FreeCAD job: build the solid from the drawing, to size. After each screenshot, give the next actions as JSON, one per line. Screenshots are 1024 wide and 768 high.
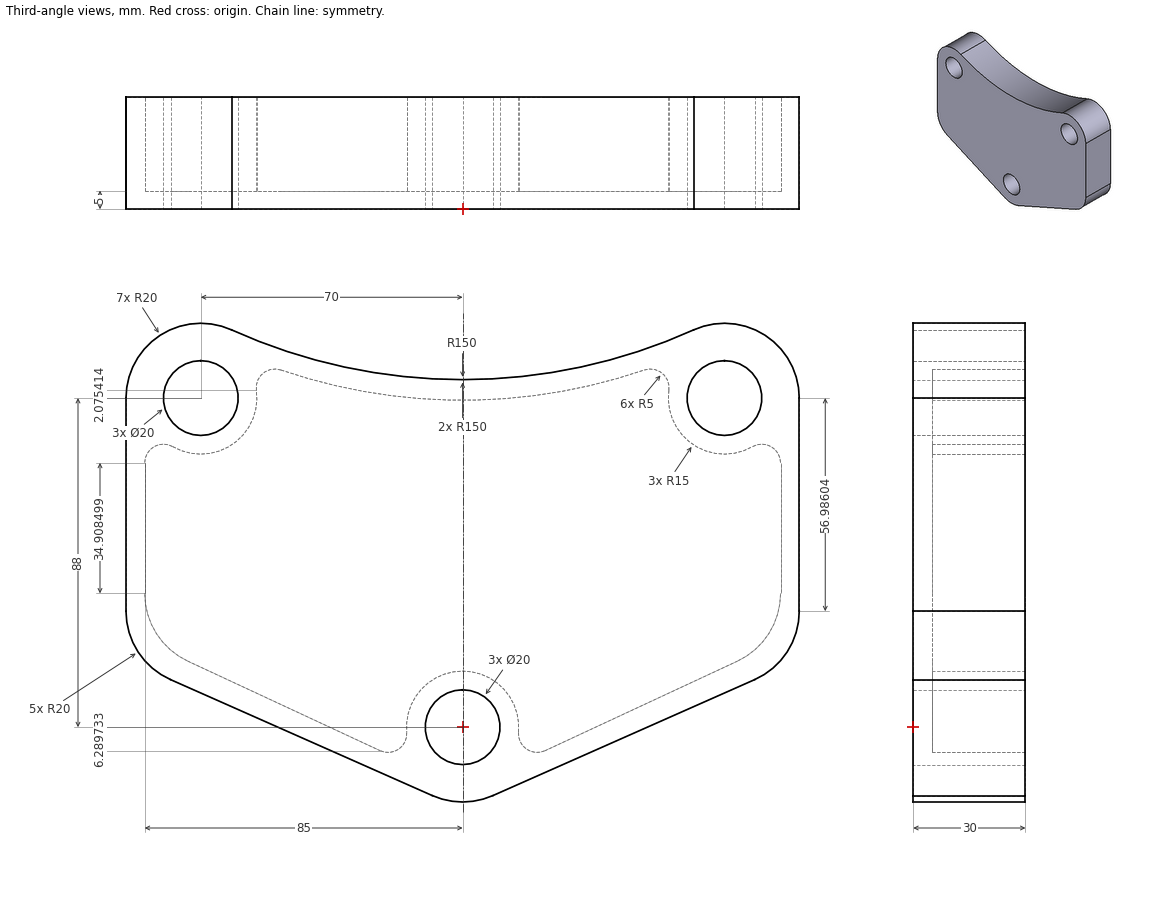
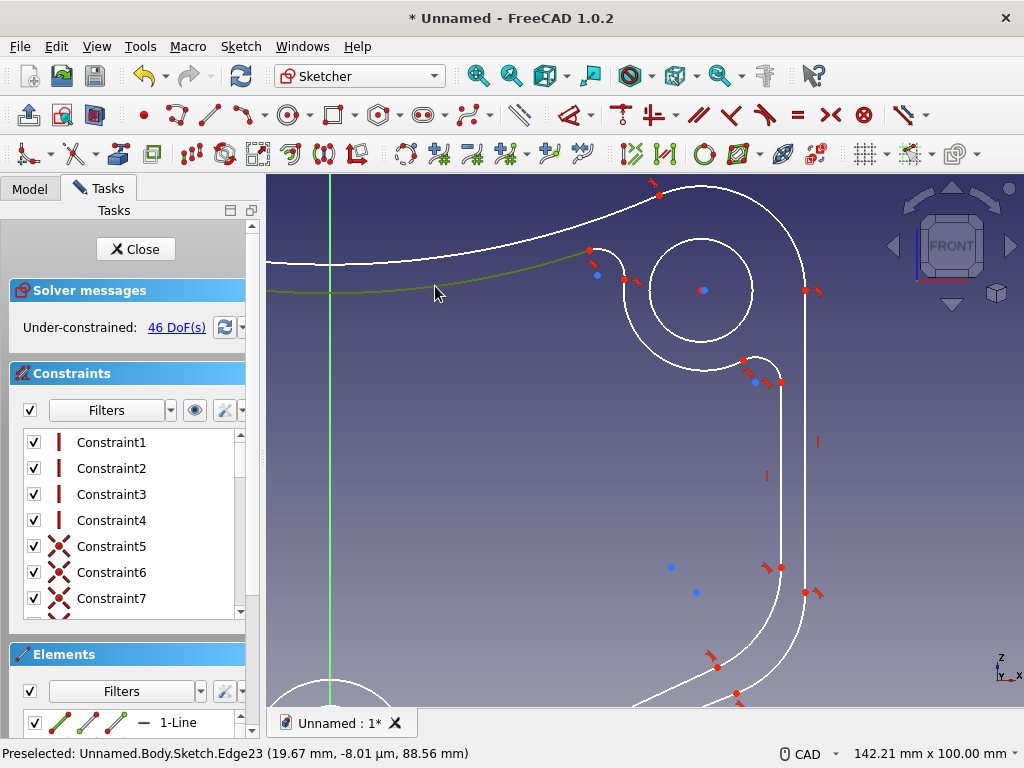
{"action": "scroll", "coordinate": [777, 369], "scroll_direction": "down", "scroll_amount": 4}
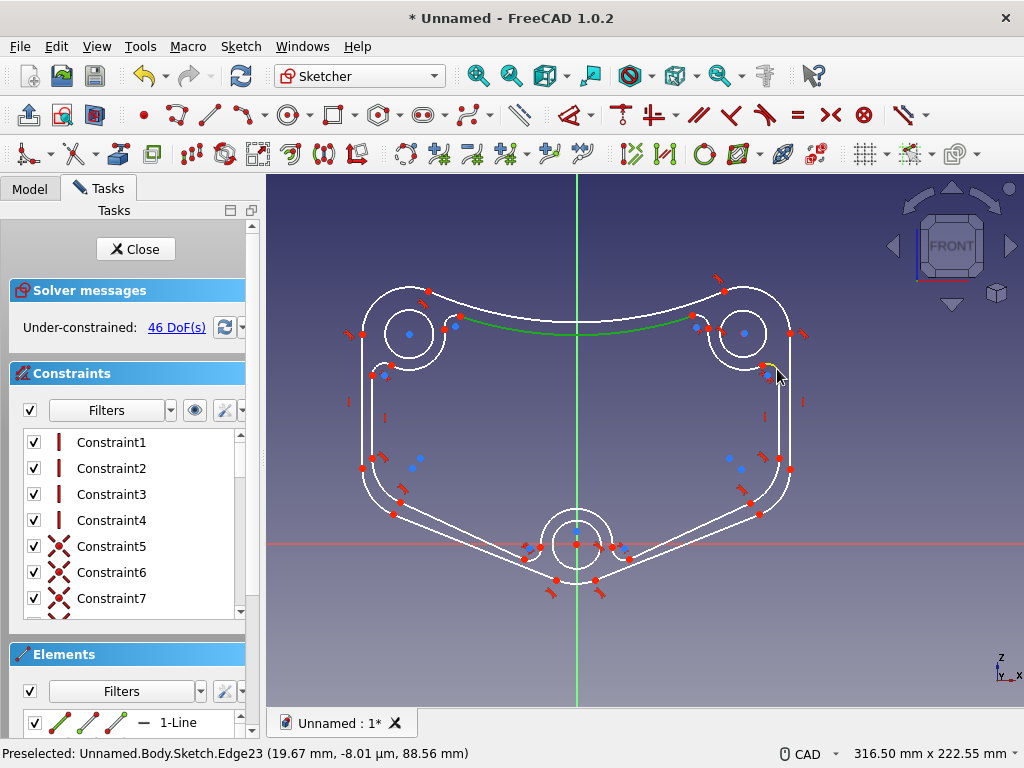
{"action": "scroll", "coordinate": [453, 316], "scroll_direction": "up", "scroll_amount": 4}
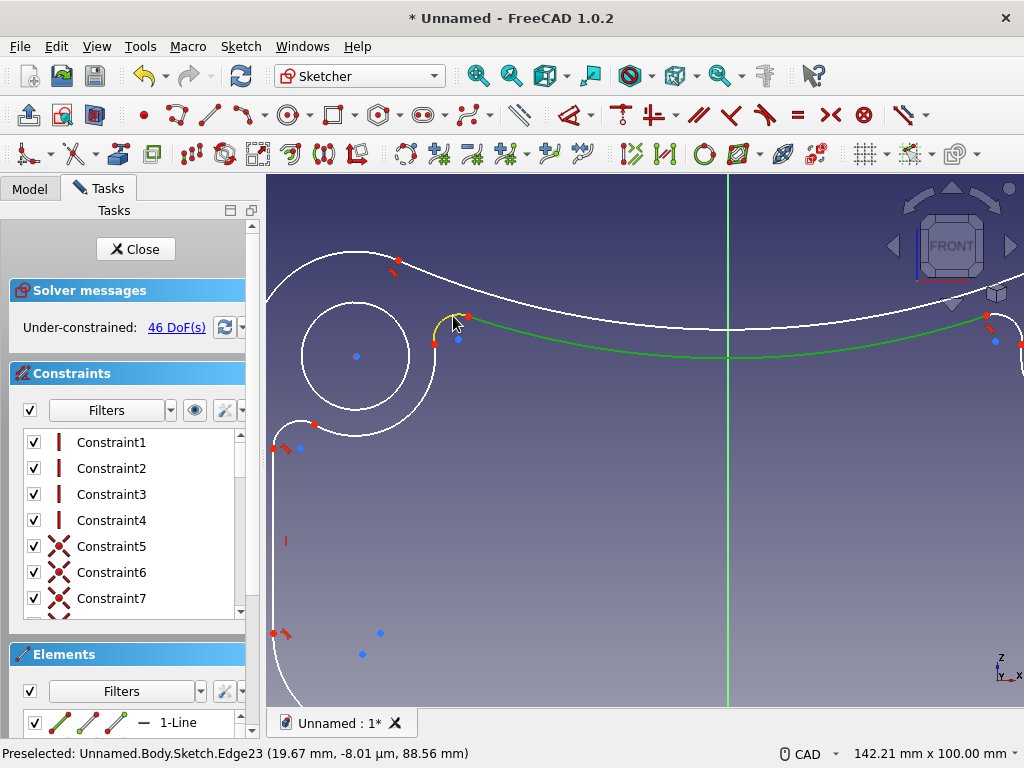
{"action": "left_click", "coordinate": [453, 315]}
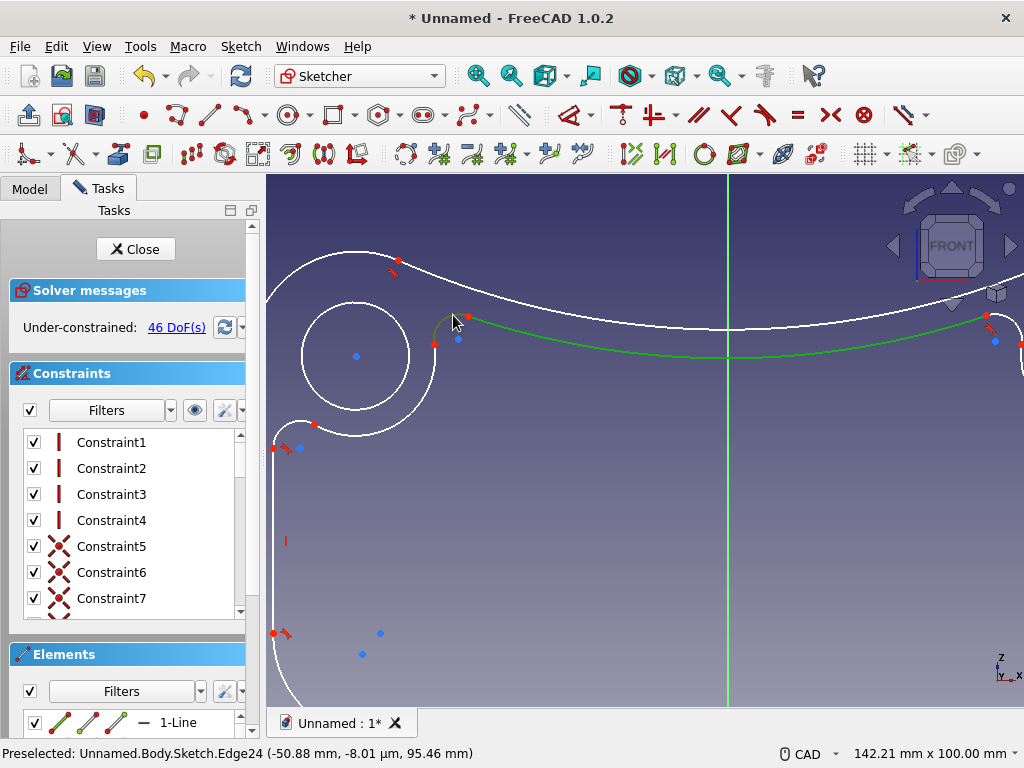
{"action": "key", "text": "t"}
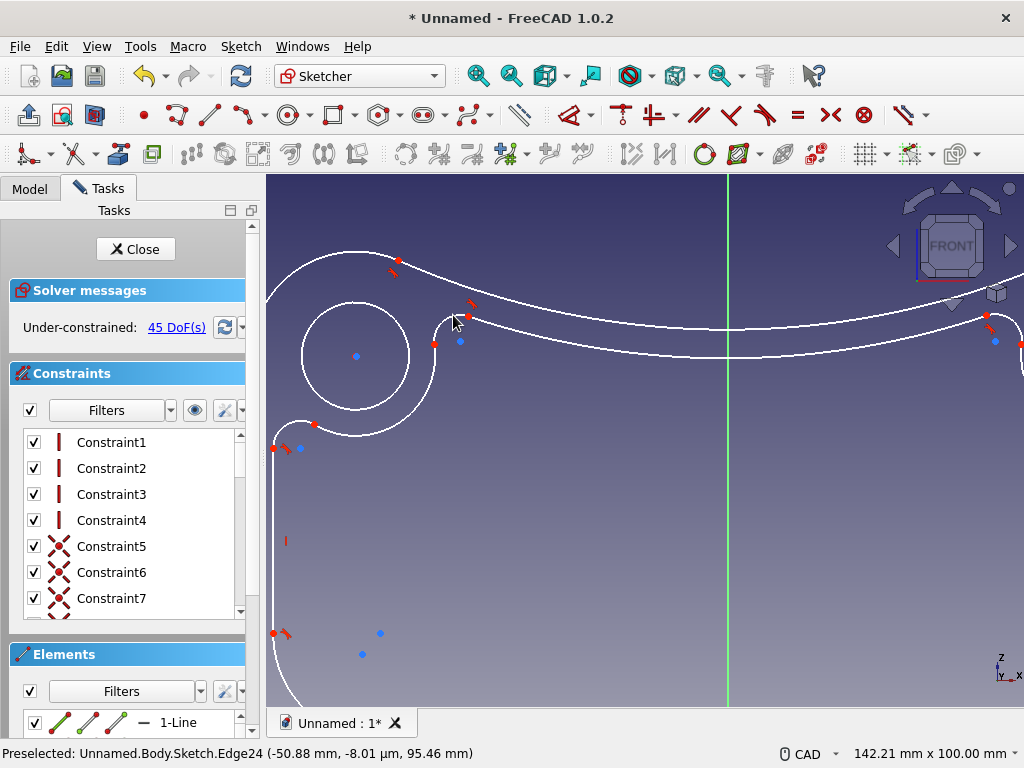
{"action": "left_click", "coordinate": [453, 316]}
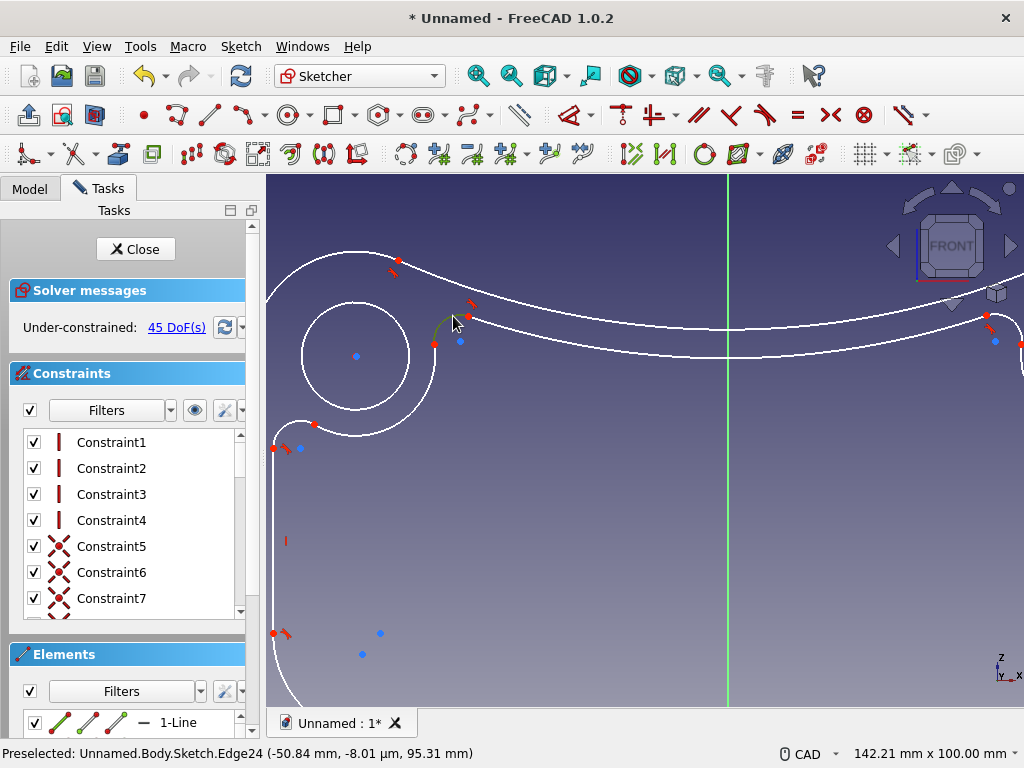
{"action": "left_click", "coordinate": [367, 435]}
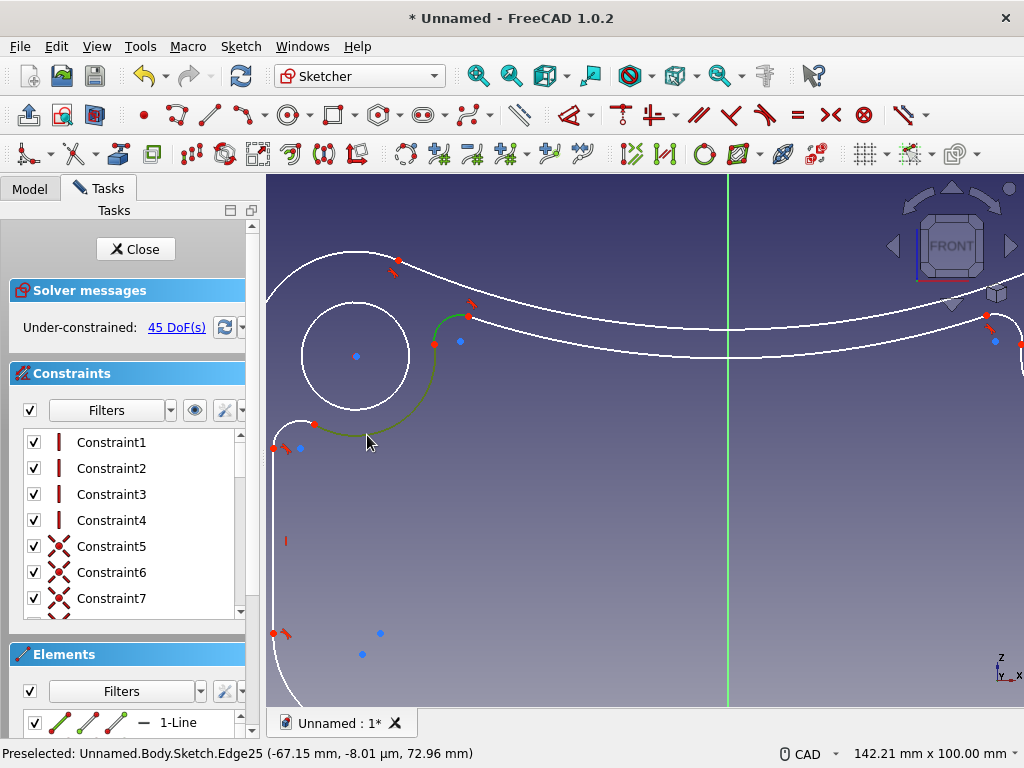
{"action": "left_click", "coordinate": [765, 116]}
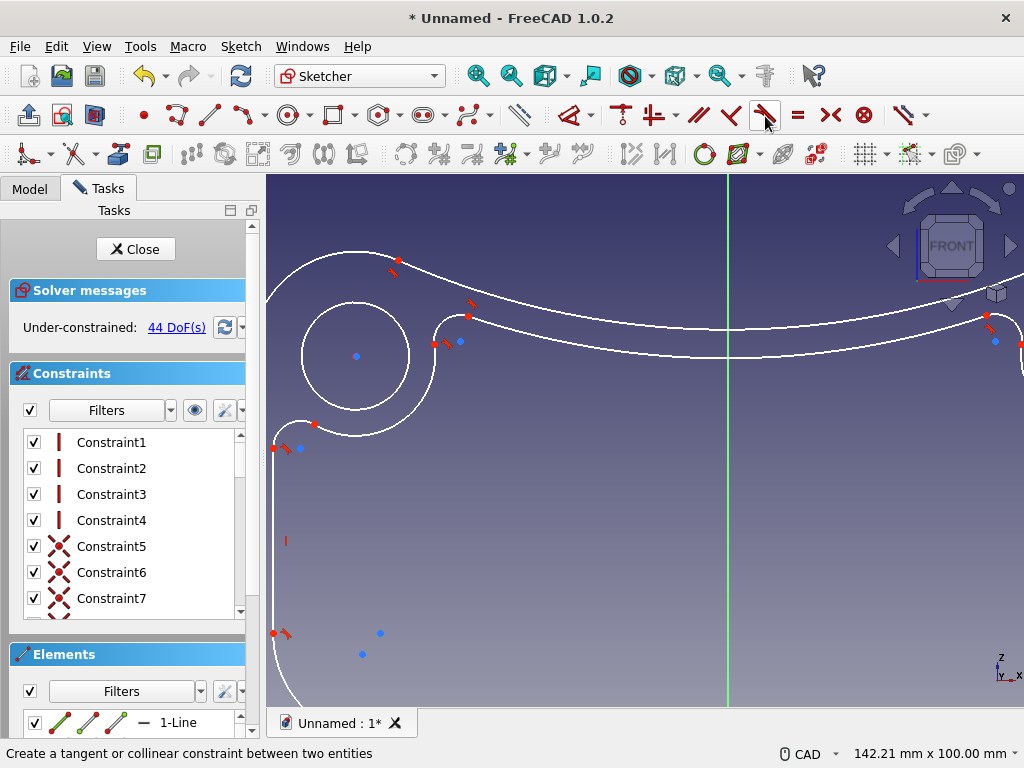
{"action": "left_click", "coordinate": [367, 435]}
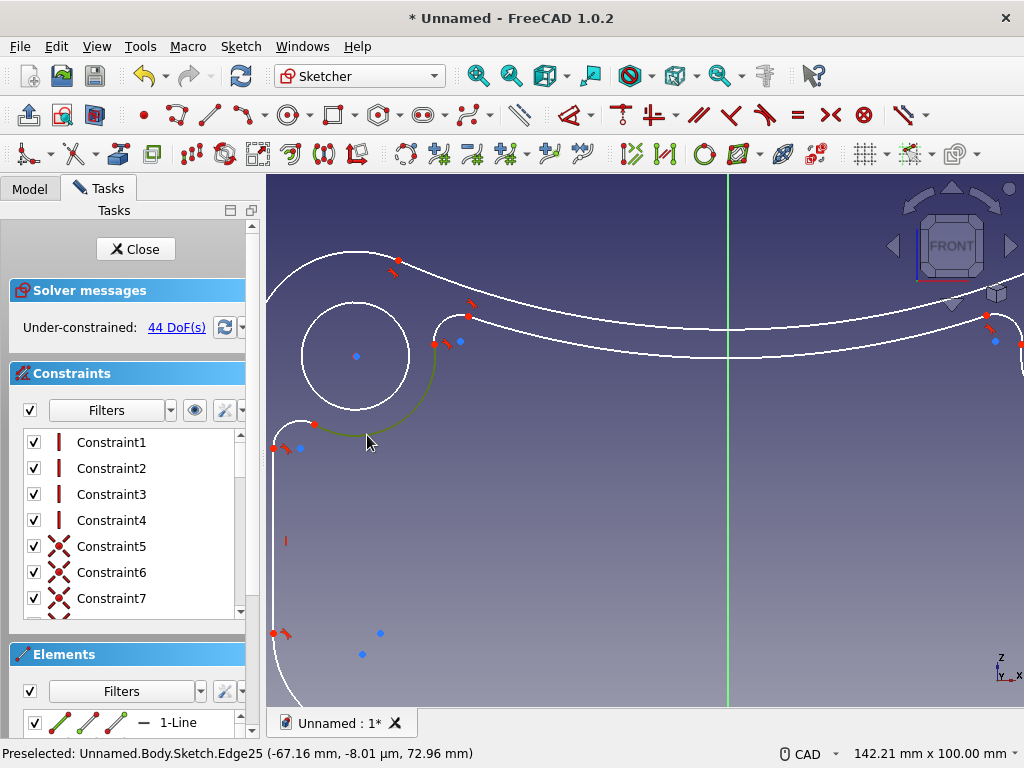
{"action": "left_click", "coordinate": [298, 421]}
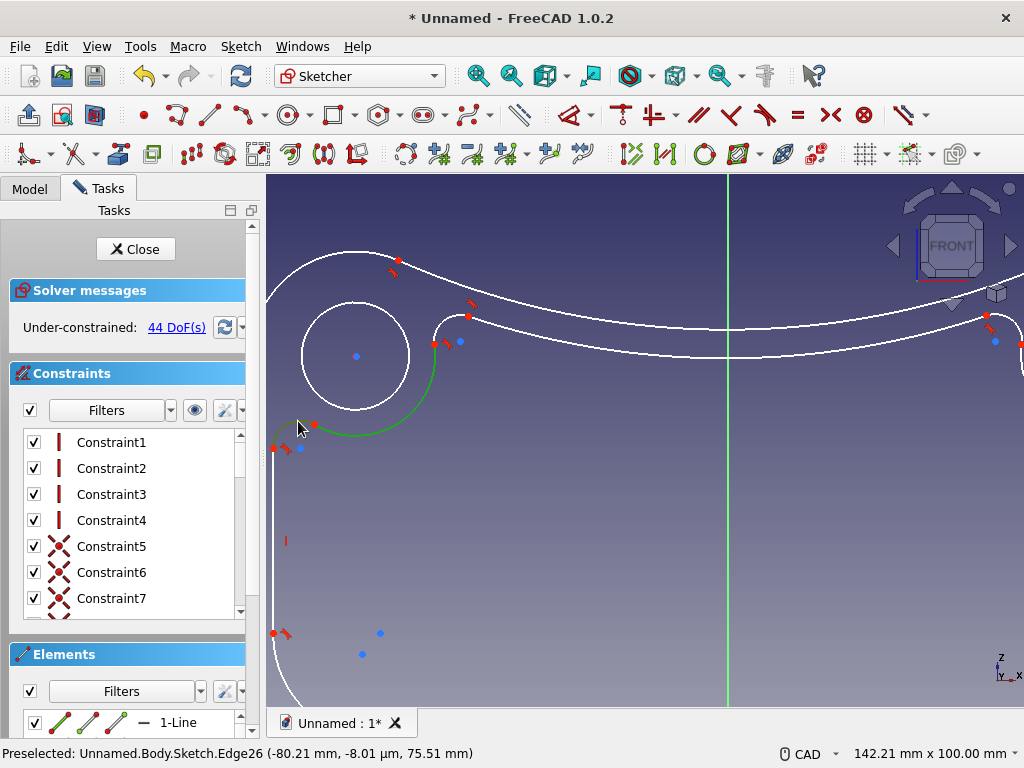
{"action": "left_click", "coordinate": [765, 116]}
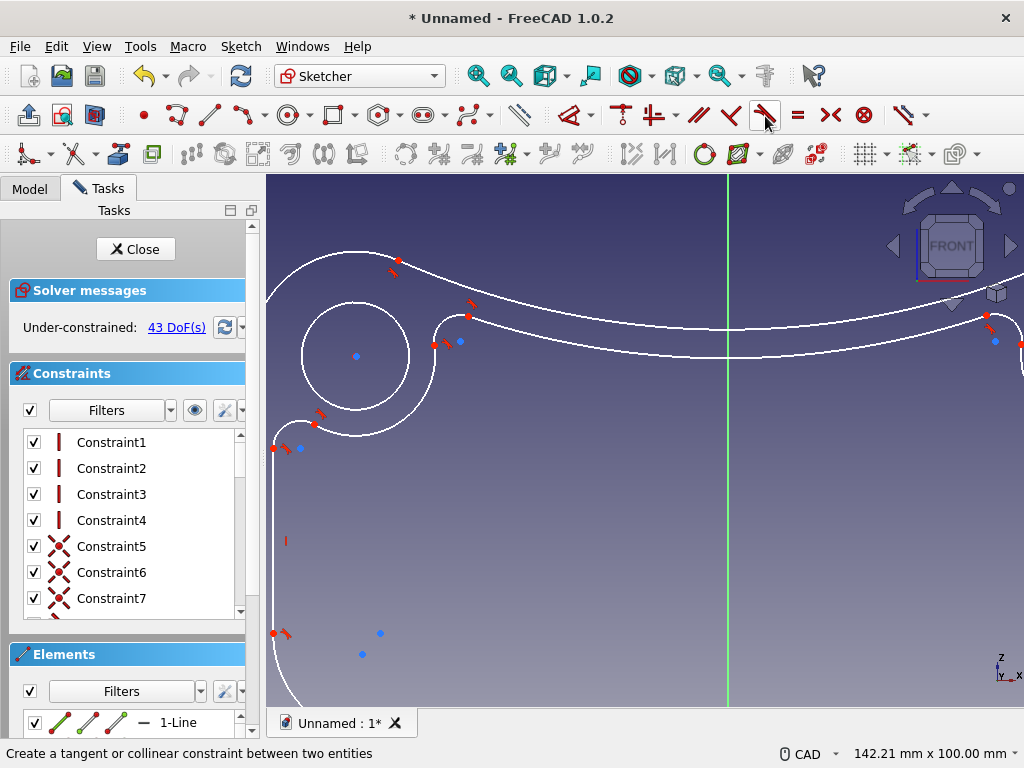
{"action": "scroll", "coordinate": [453, 316], "scroll_direction": "down", "scroll_amount": 4}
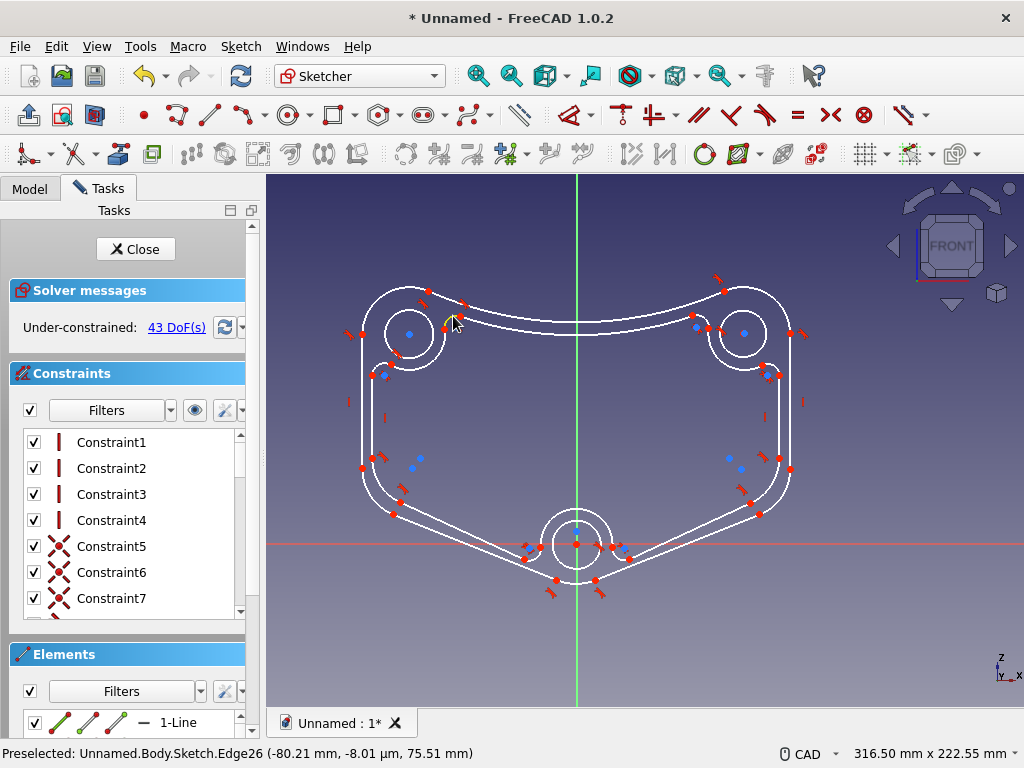
{"action": "left_click", "coordinate": [594, 528]}